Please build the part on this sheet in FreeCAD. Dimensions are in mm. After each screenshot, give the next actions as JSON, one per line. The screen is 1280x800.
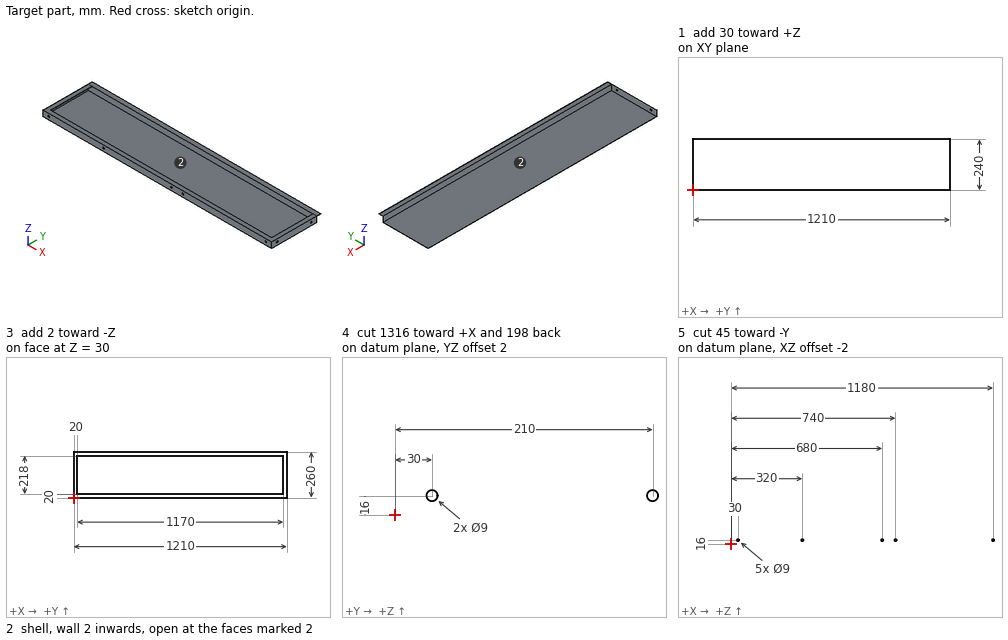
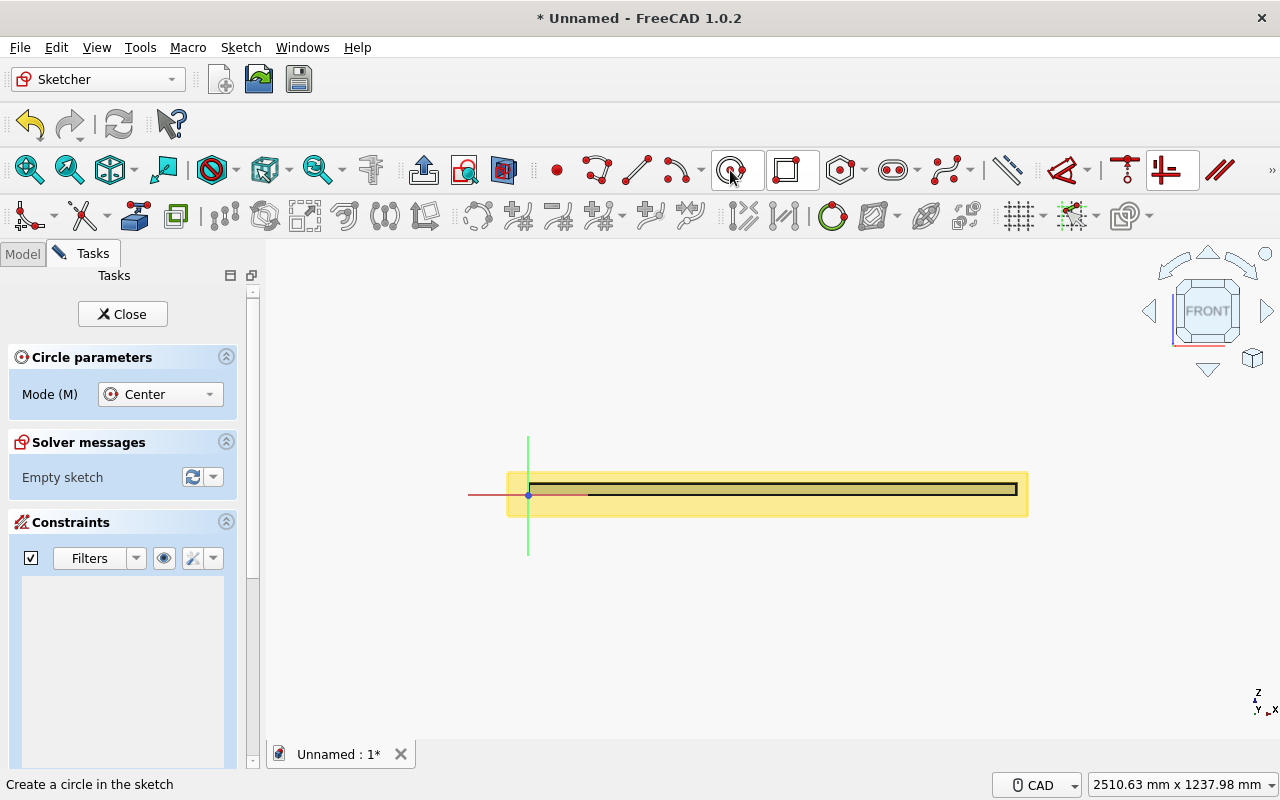
{"action": "scroll", "coordinate": [541, 489], "scroll_direction": "up", "scroll_amount": 13}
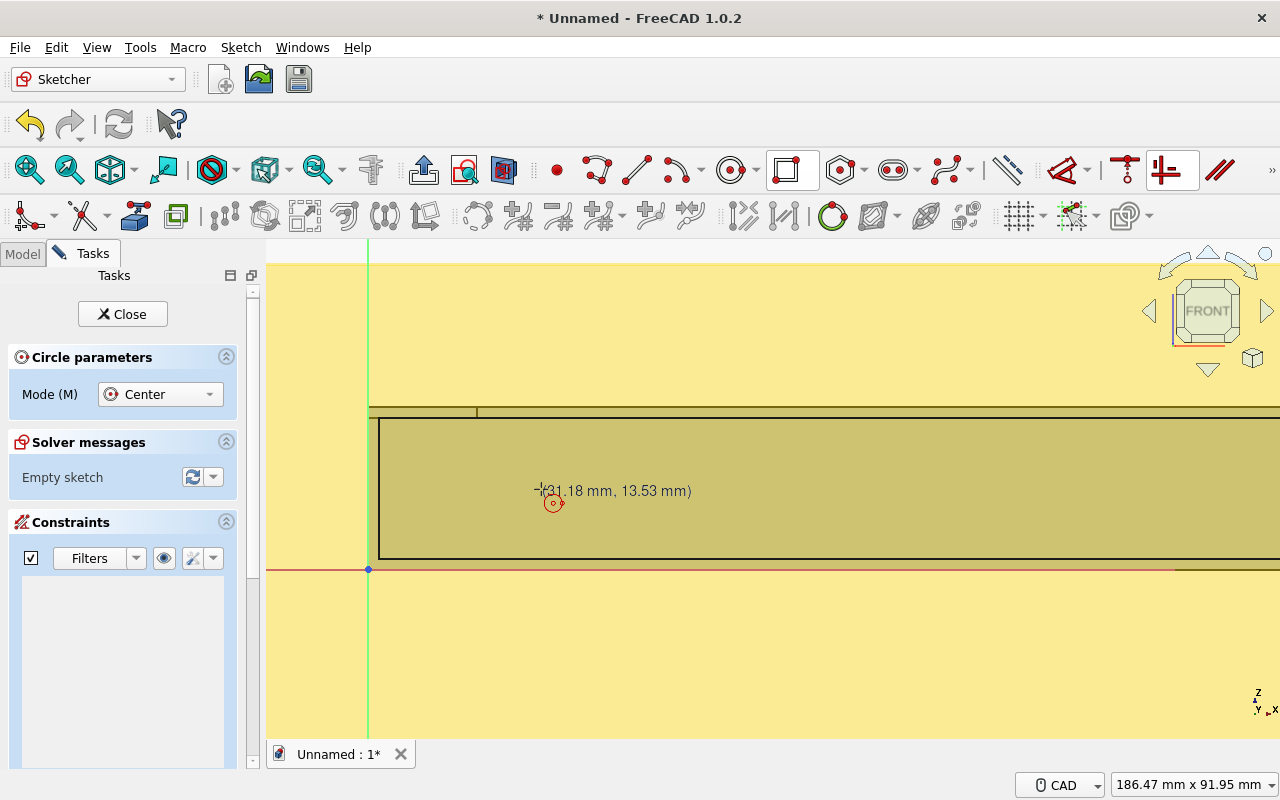
{"action": "scroll", "coordinate": [417, 486], "scroll_direction": "down", "scroll_amount": 12}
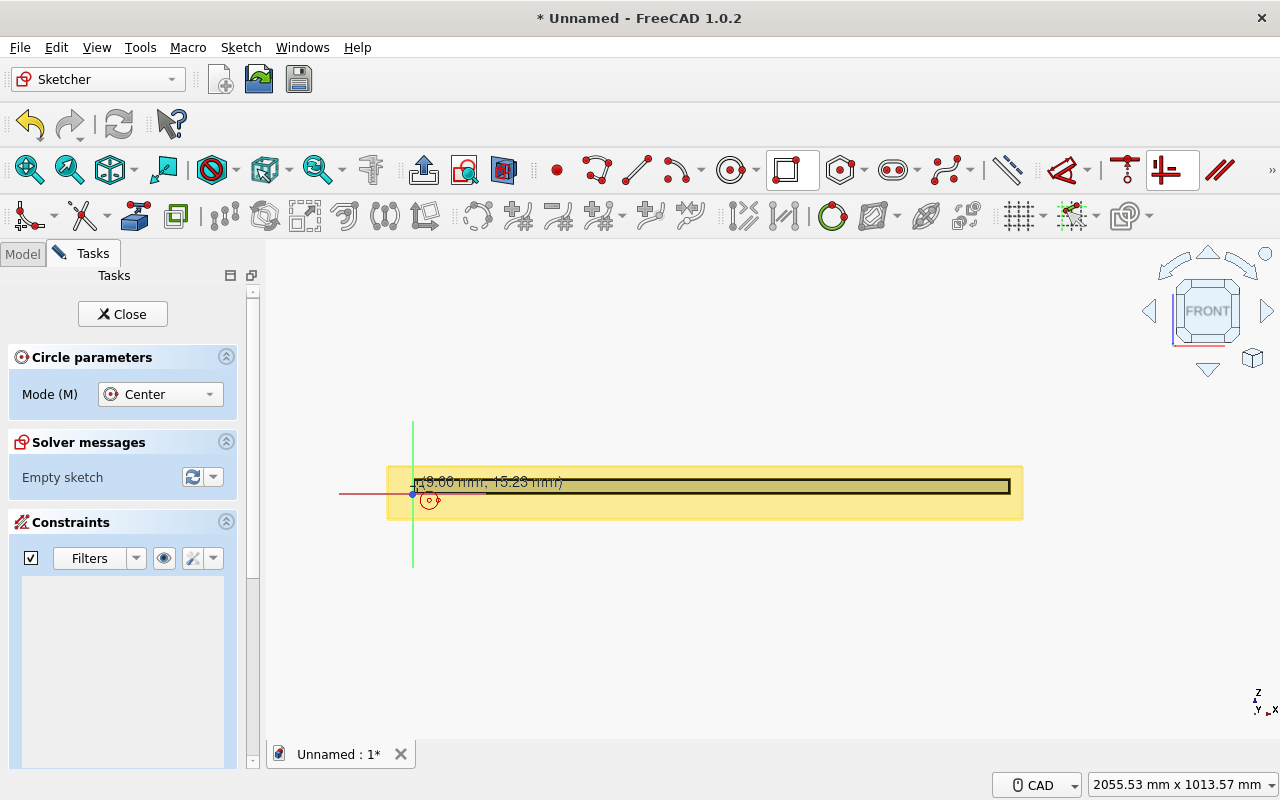
{"action": "scroll", "coordinate": [427, 486], "scroll_direction": "up", "scroll_amount": 4}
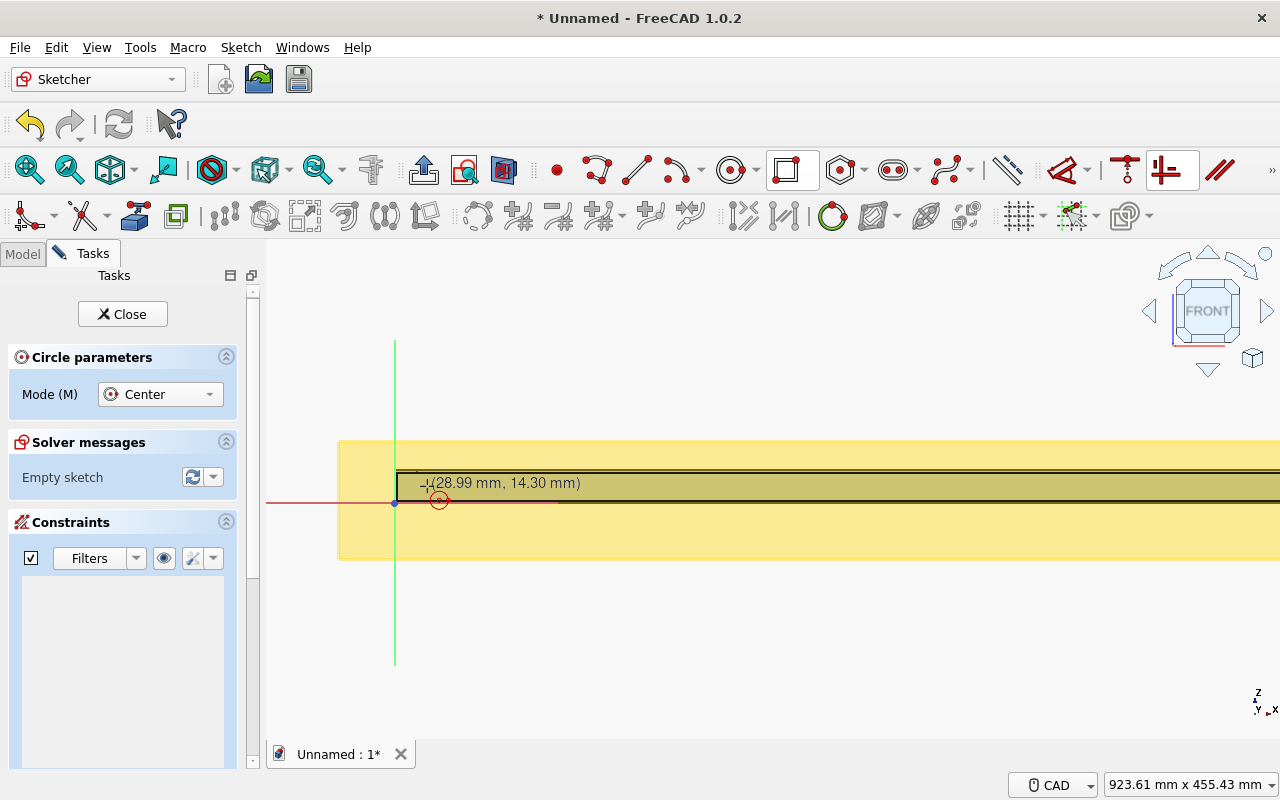
{"action": "left_click", "coordinate": [428, 486]}
{"action": "mouse_move", "coordinate": [431, 482]}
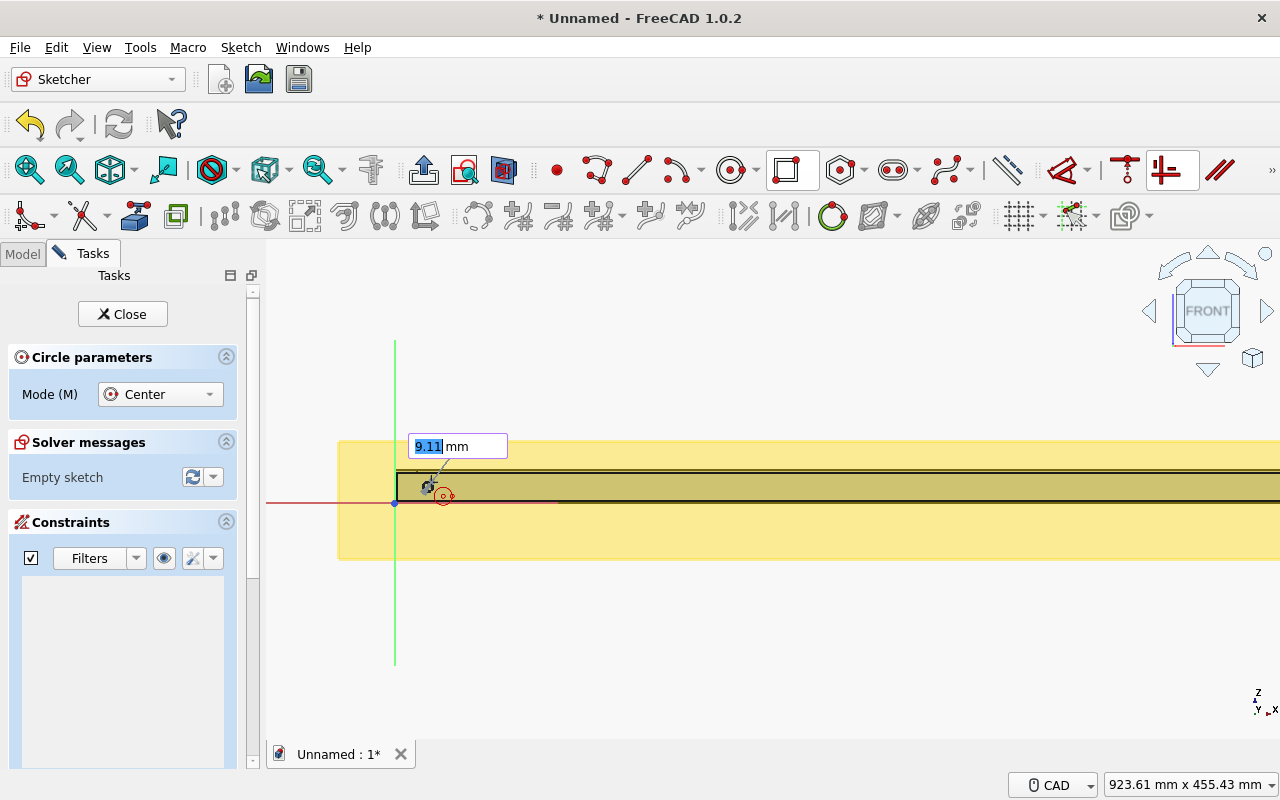
{"action": "type", "text": "9"}
{"action": "key", "text": "Return"}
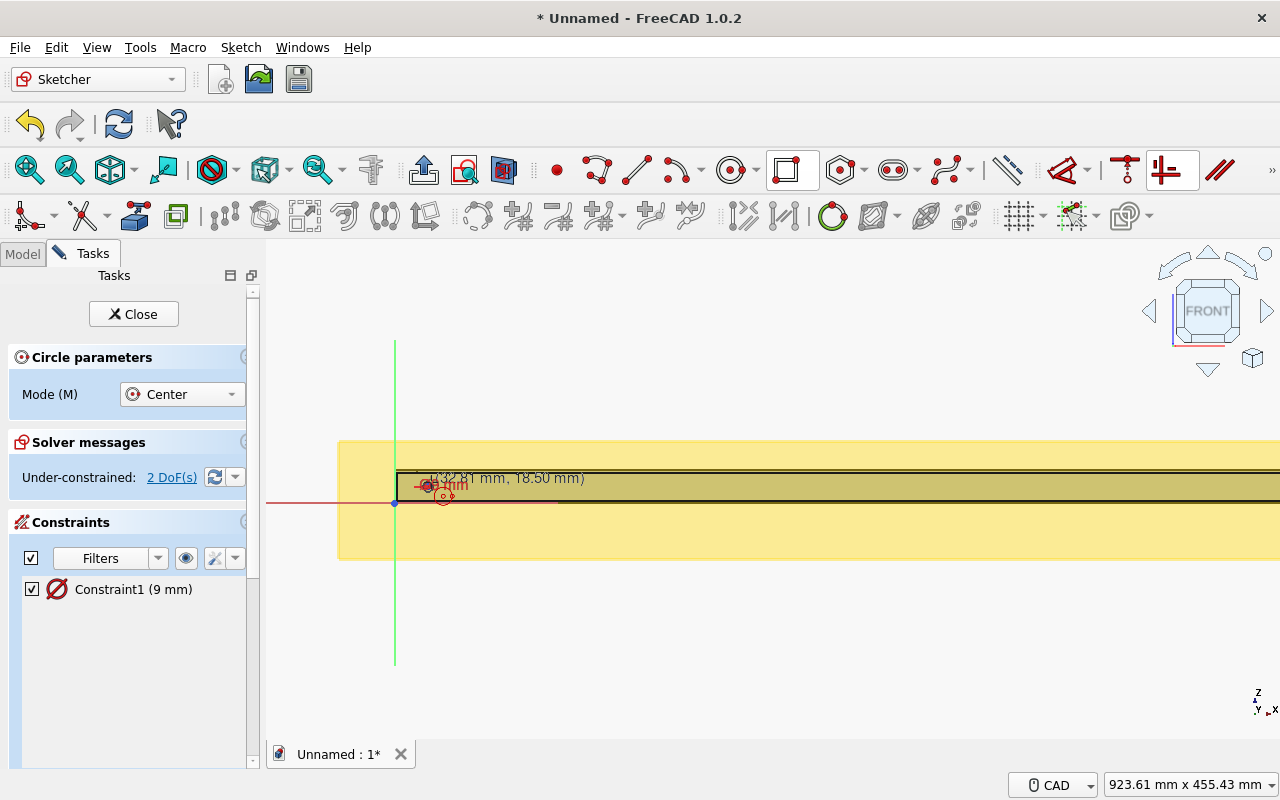
{"action": "scroll", "coordinate": [427, 487], "scroll_direction": "down", "scroll_amount": 4}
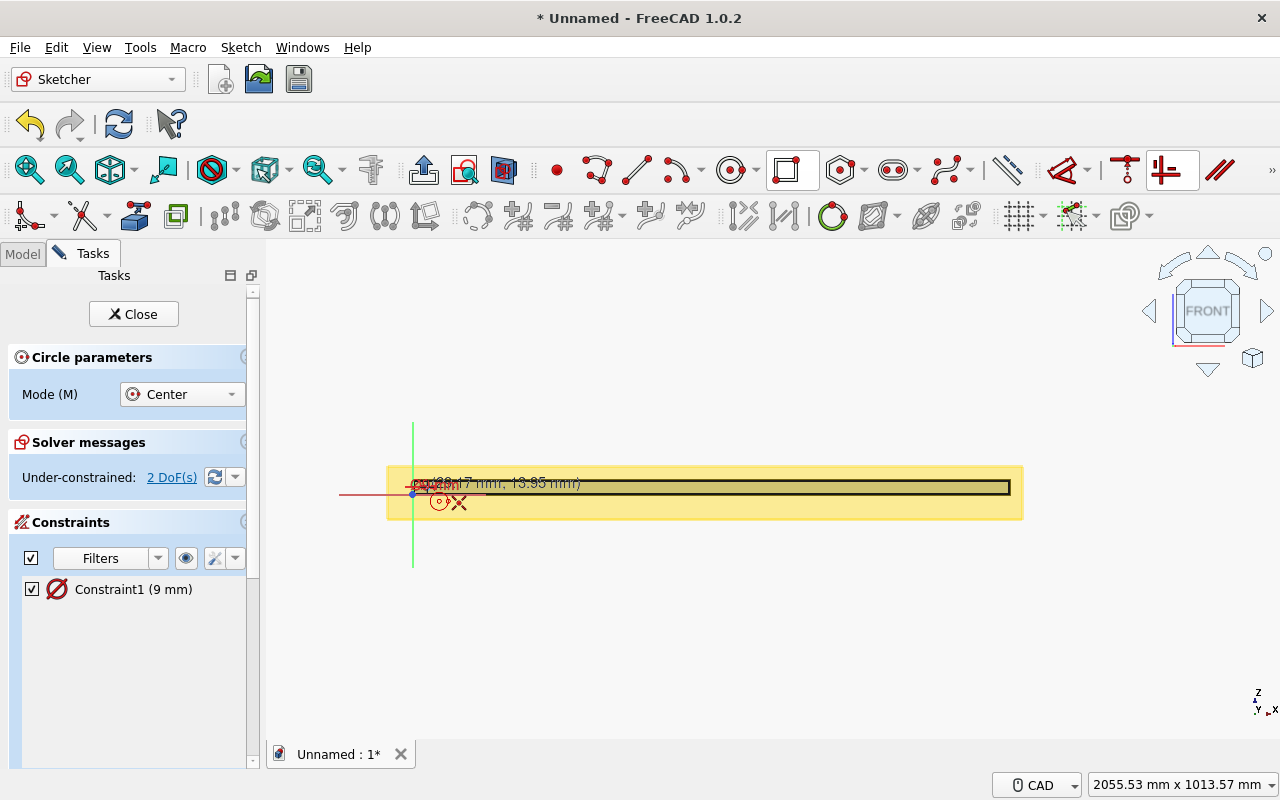
{"action": "scroll", "coordinate": [995, 487], "scroll_direction": "up", "scroll_amount": 12}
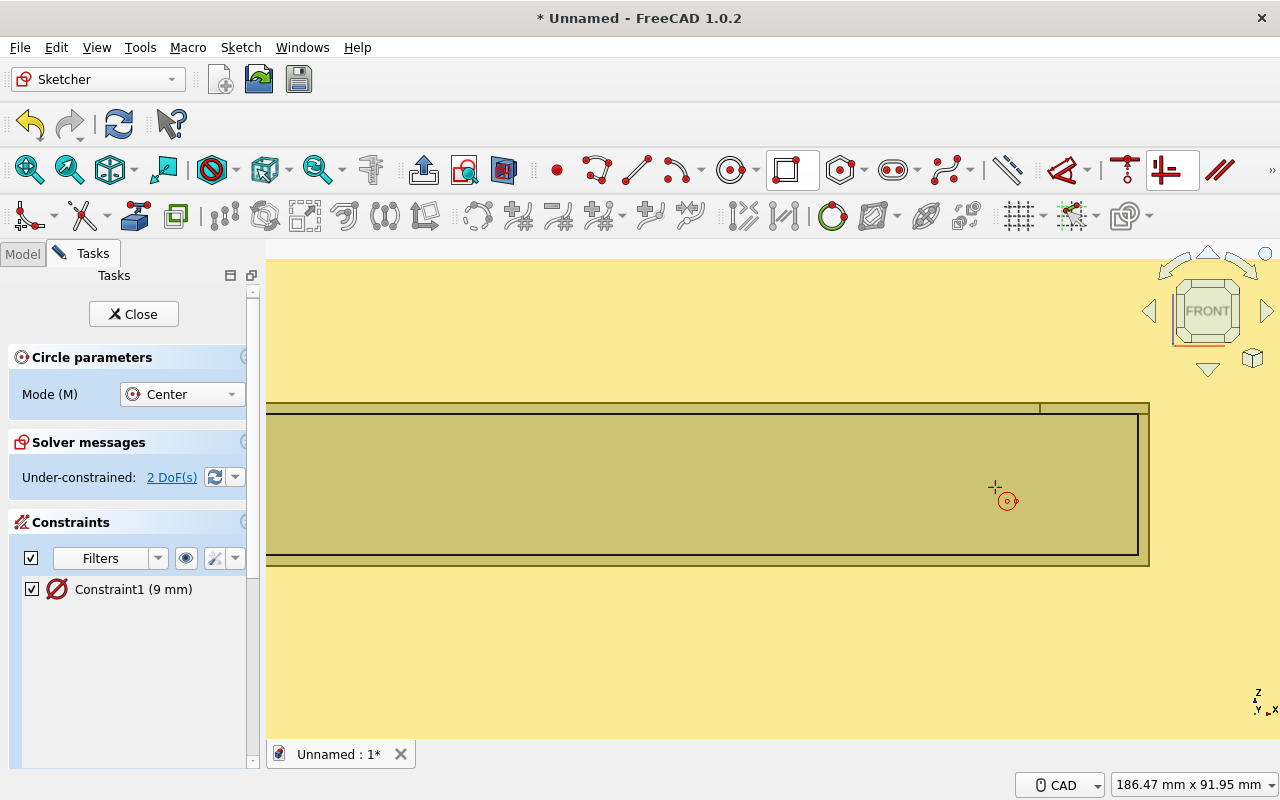
{"action": "scroll", "coordinate": [995, 487], "scroll_direction": "down", "scroll_amount": 12}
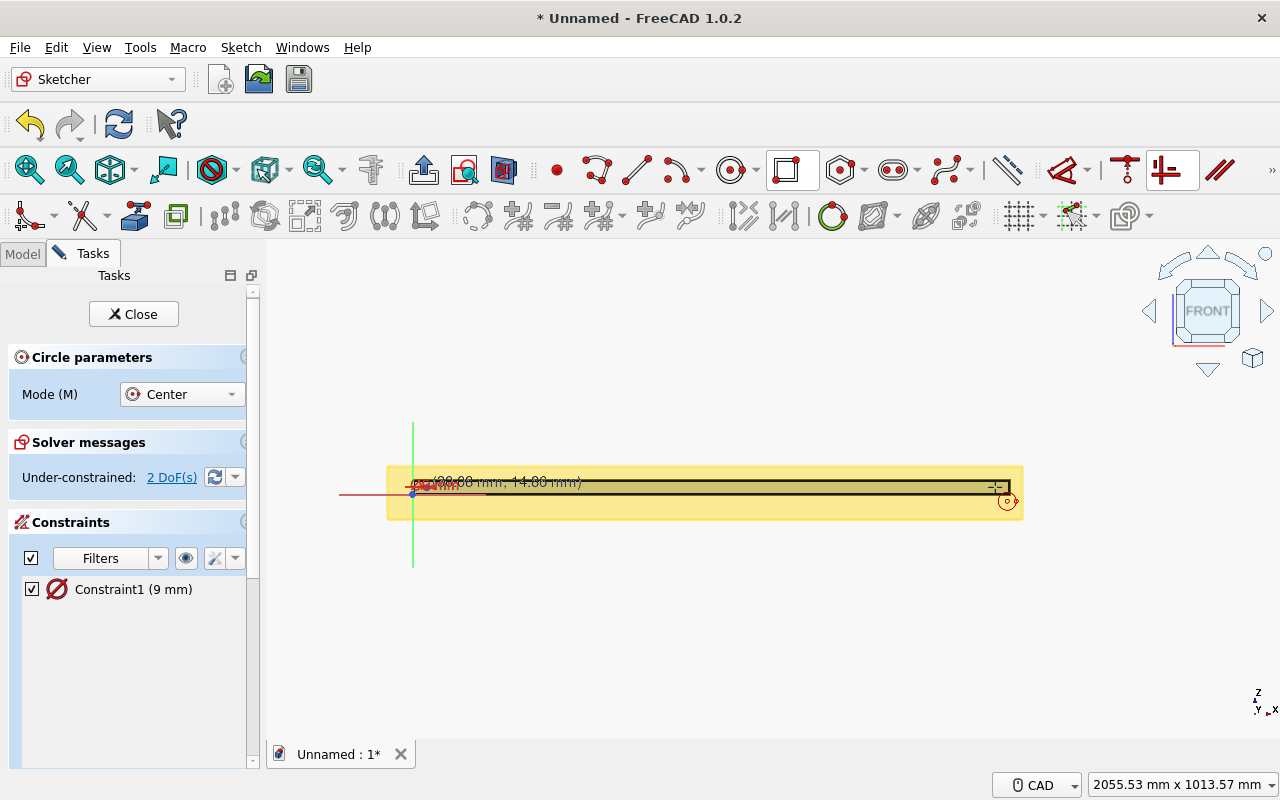
{"action": "scroll", "coordinate": [995, 487], "scroll_direction": "up", "scroll_amount": 4}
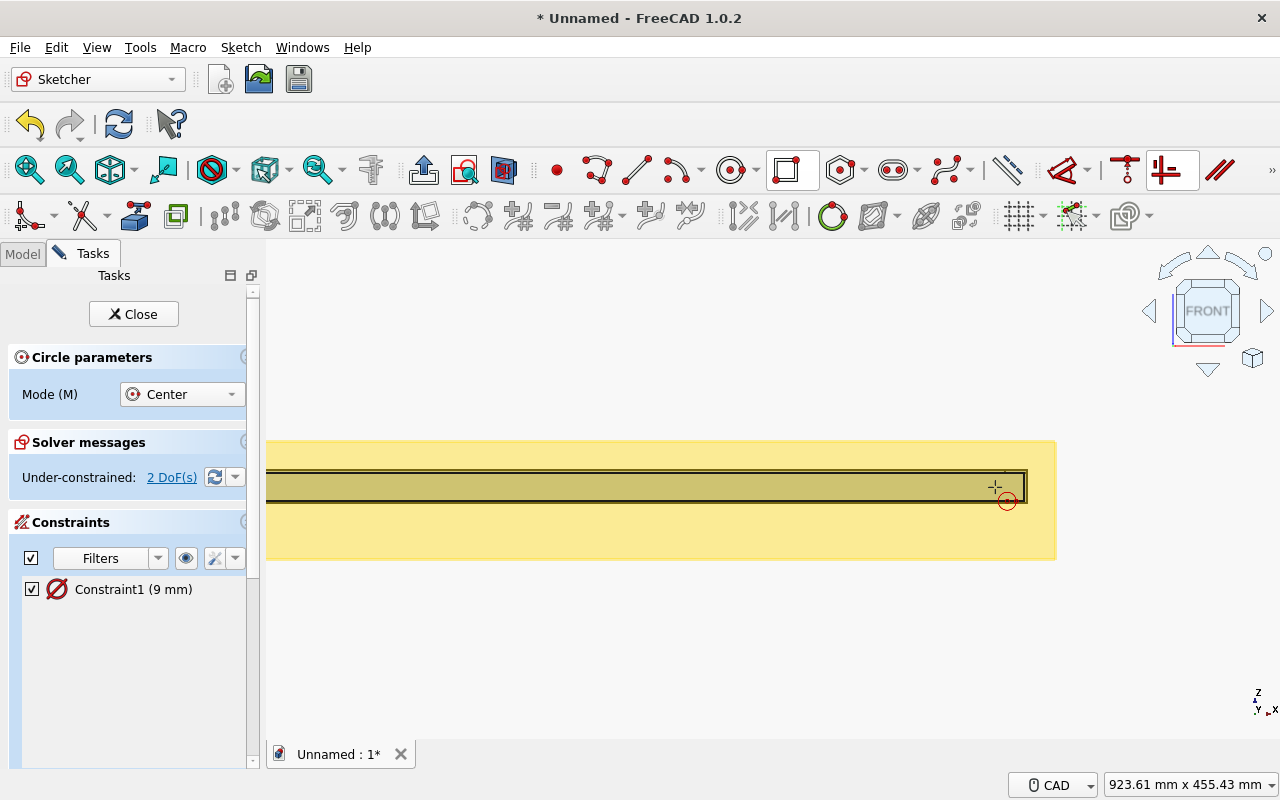
{"action": "left_click", "coordinate": [994, 486]}
{"action": "mouse_move", "coordinate": [997, 482]}